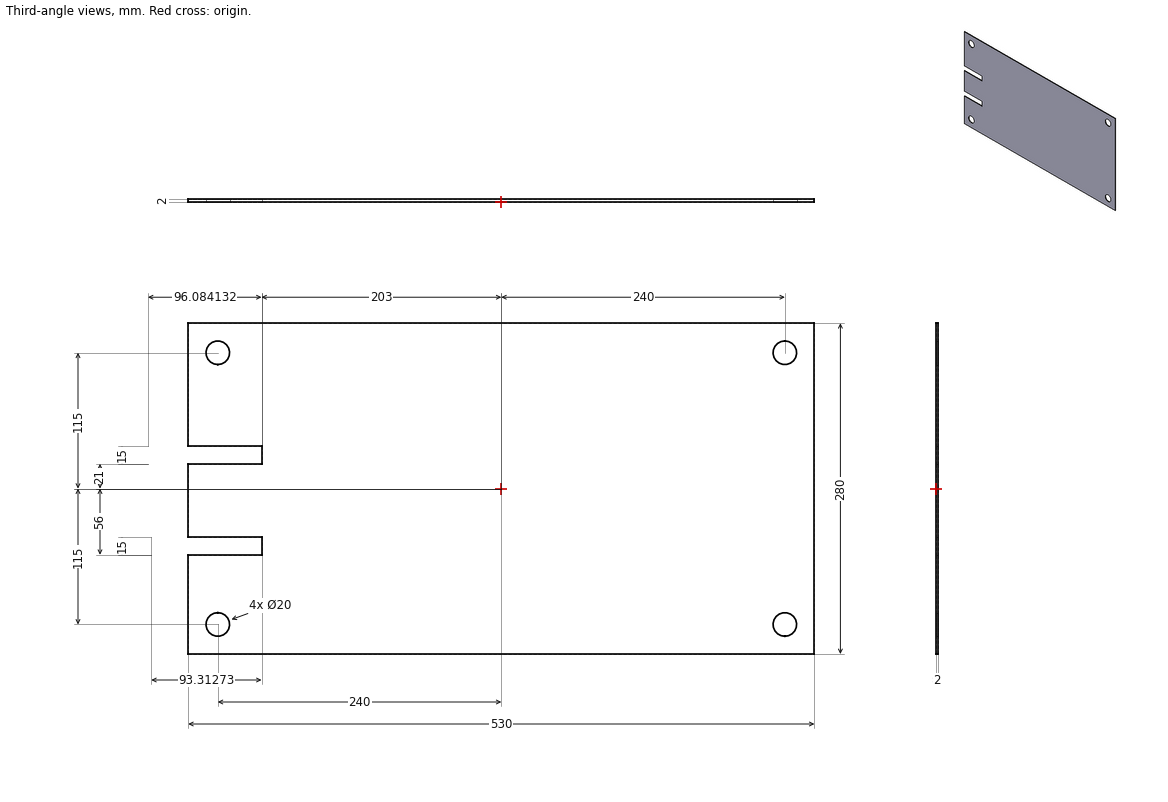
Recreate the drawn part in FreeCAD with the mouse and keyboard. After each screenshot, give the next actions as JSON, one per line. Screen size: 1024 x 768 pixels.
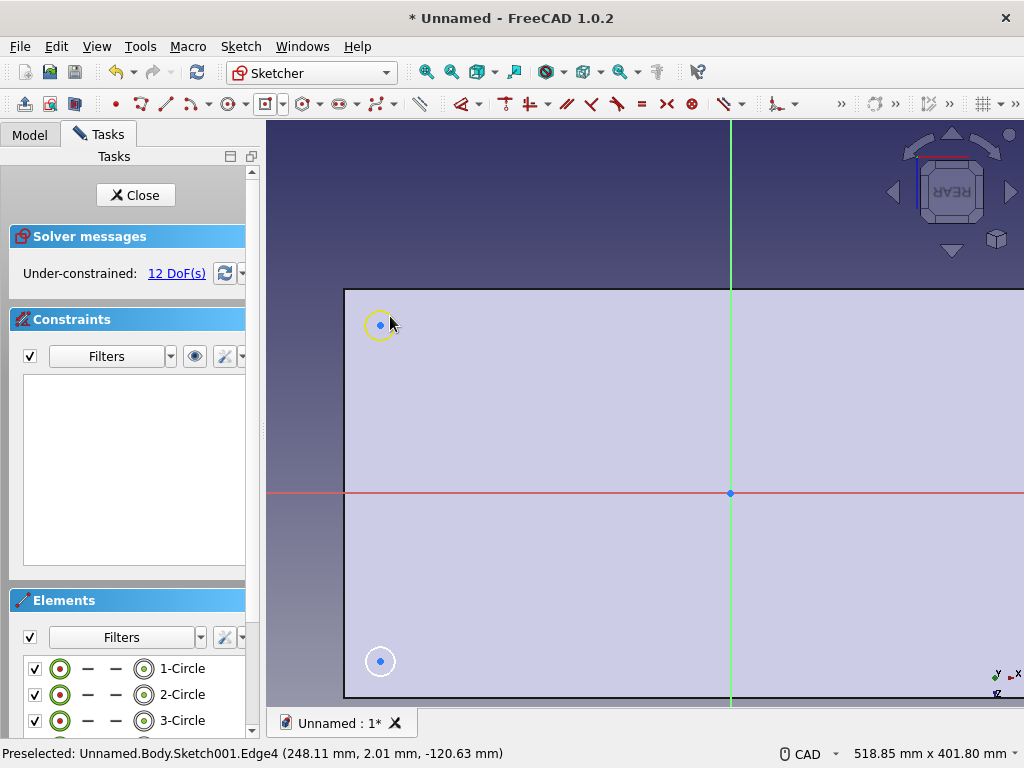
{"action": "left_click", "coordinate": [390, 315]}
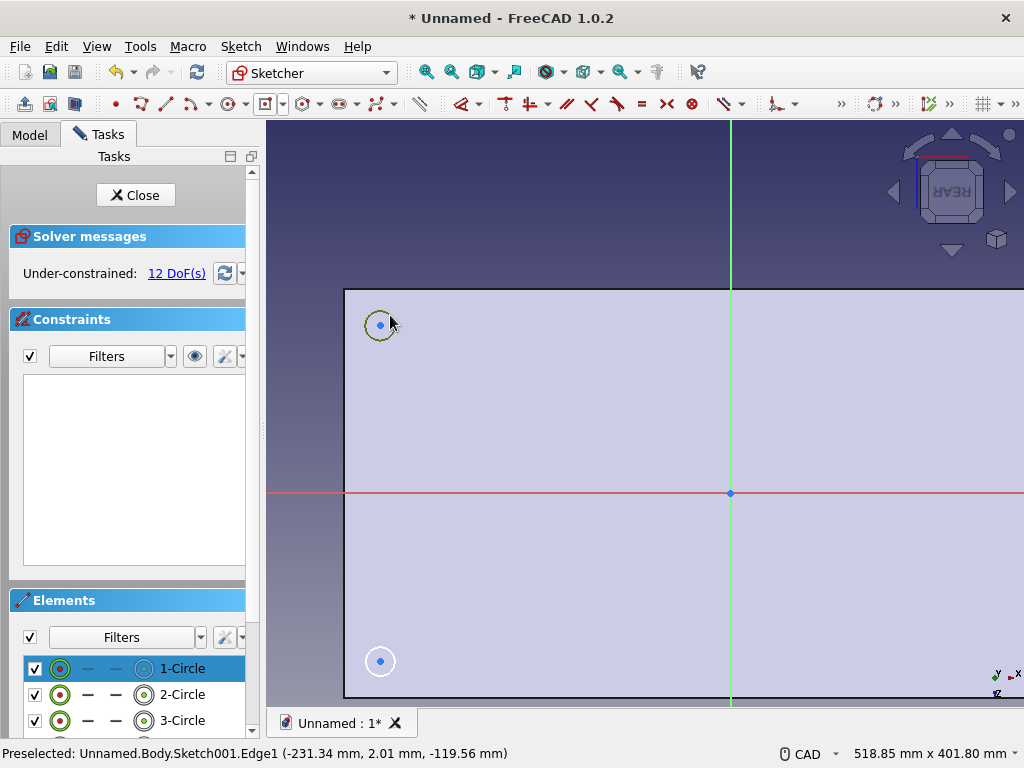
{"action": "left_click", "coordinate": [391, 651]}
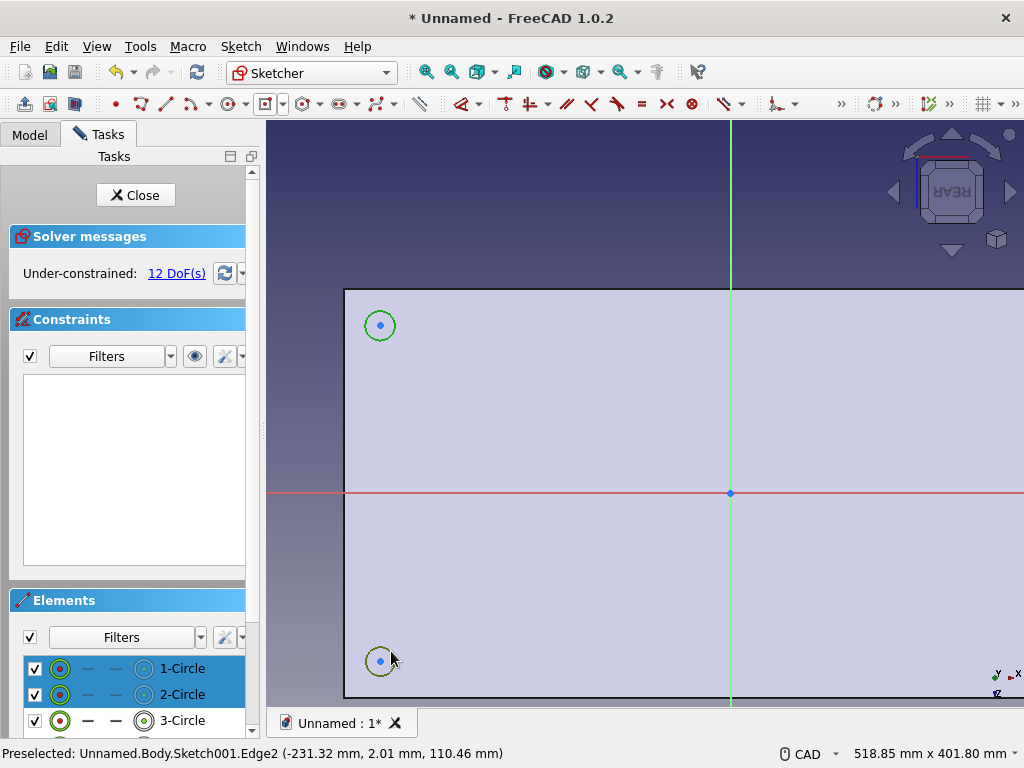
{"action": "scroll", "coordinate": [389, 316], "scroll_direction": "down", "scroll_amount": 3}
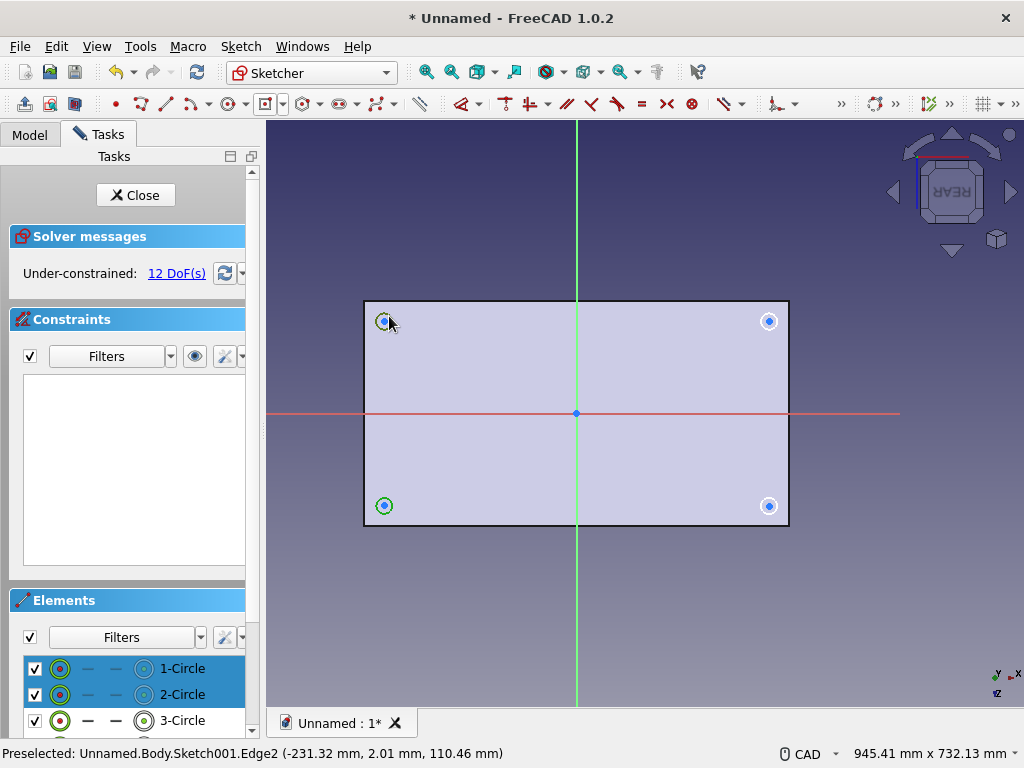
{"action": "scroll", "coordinate": [775, 500], "scroll_direction": "up", "scroll_amount": 3}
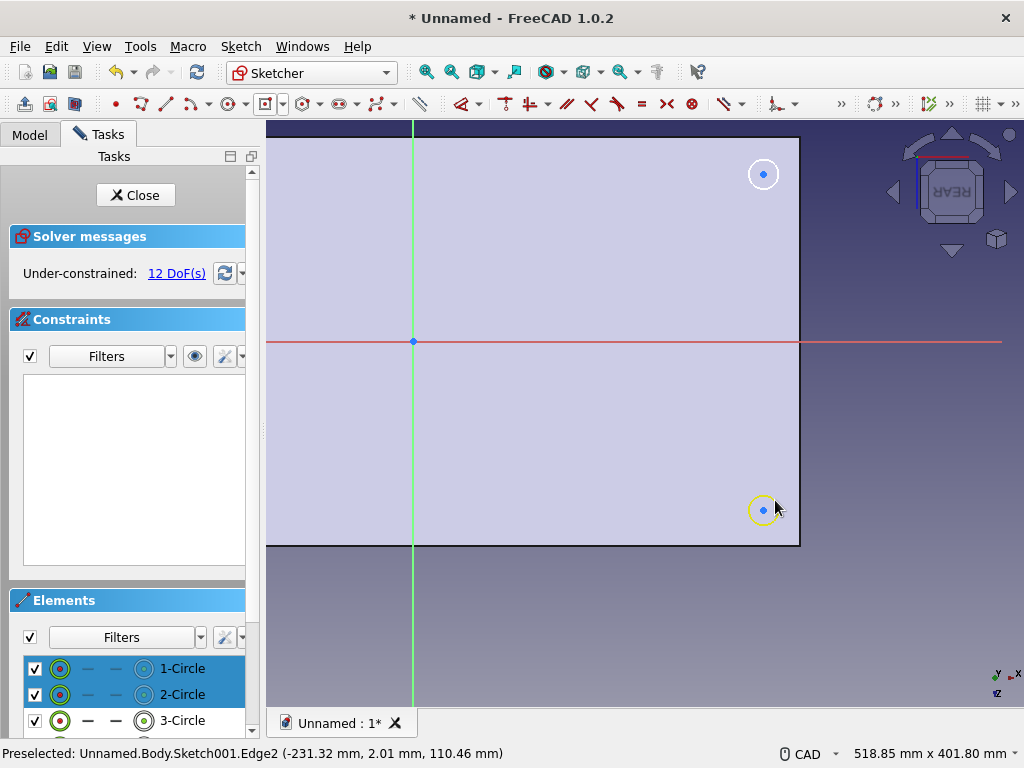
{"action": "left_click", "coordinate": [774, 500]}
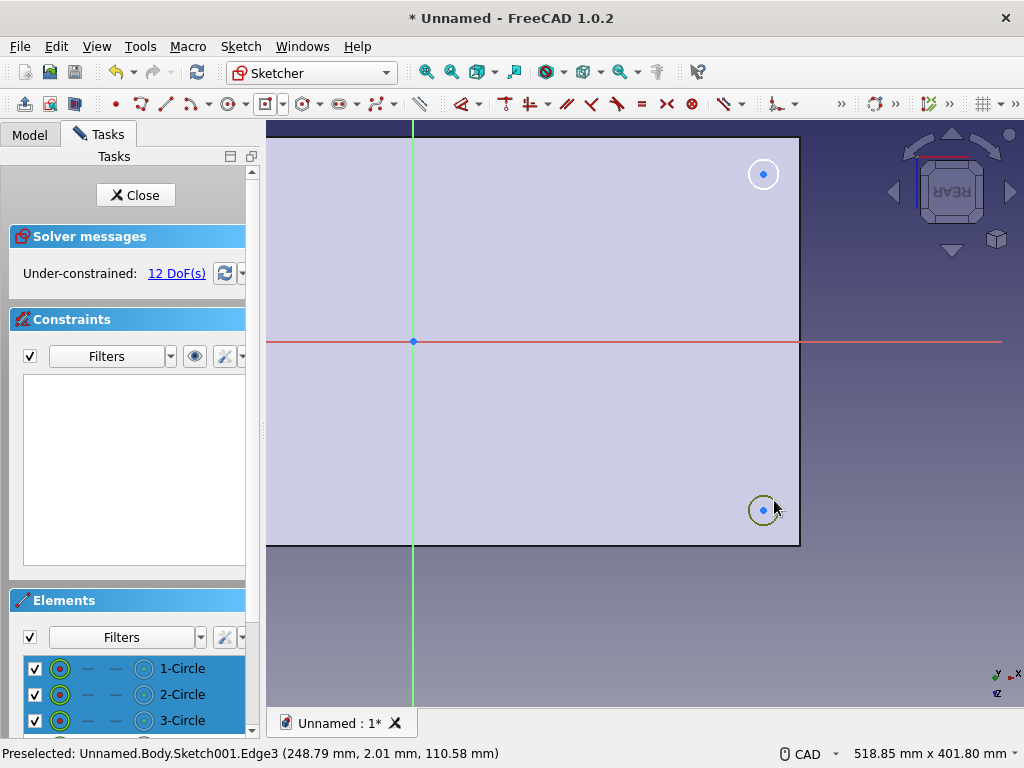
{"action": "left_click", "coordinate": [774, 164]}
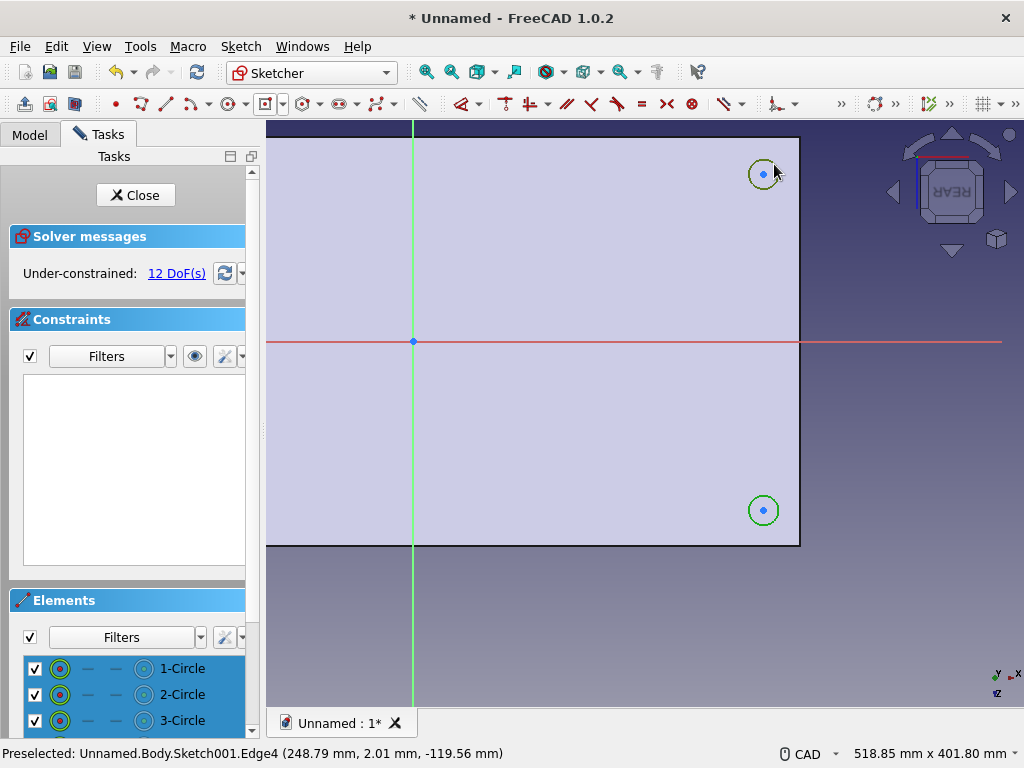
{"action": "left_click", "coordinate": [642, 104]}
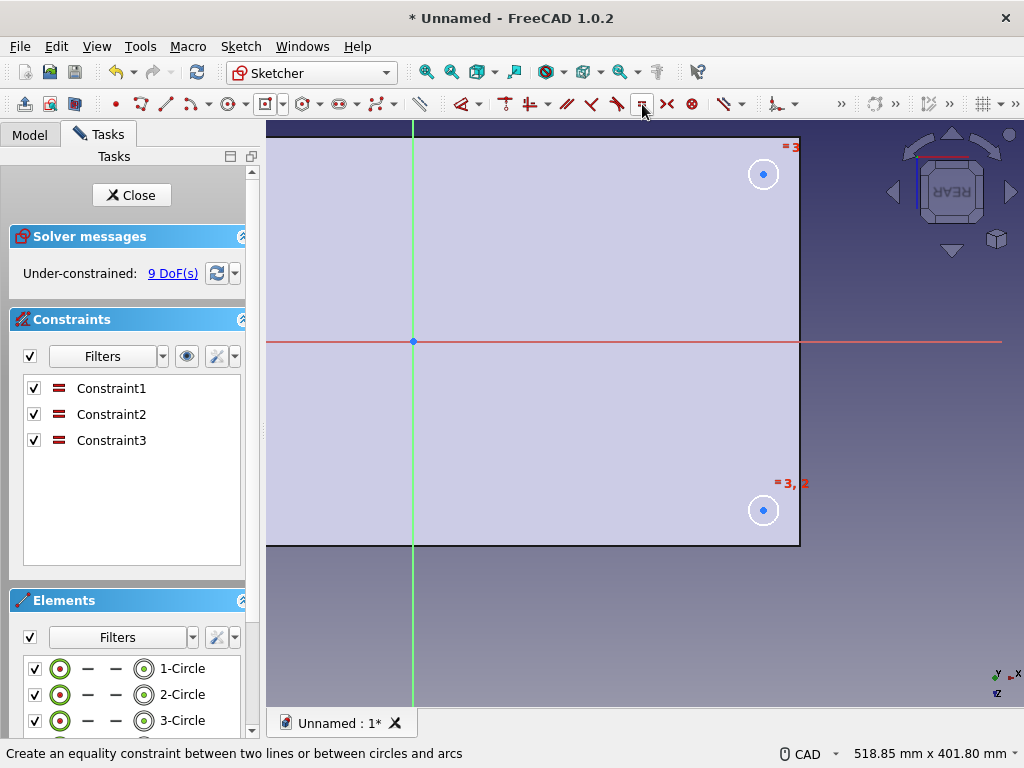
{"action": "scroll", "coordinate": [775, 501], "scroll_direction": "down", "scroll_amount": 3}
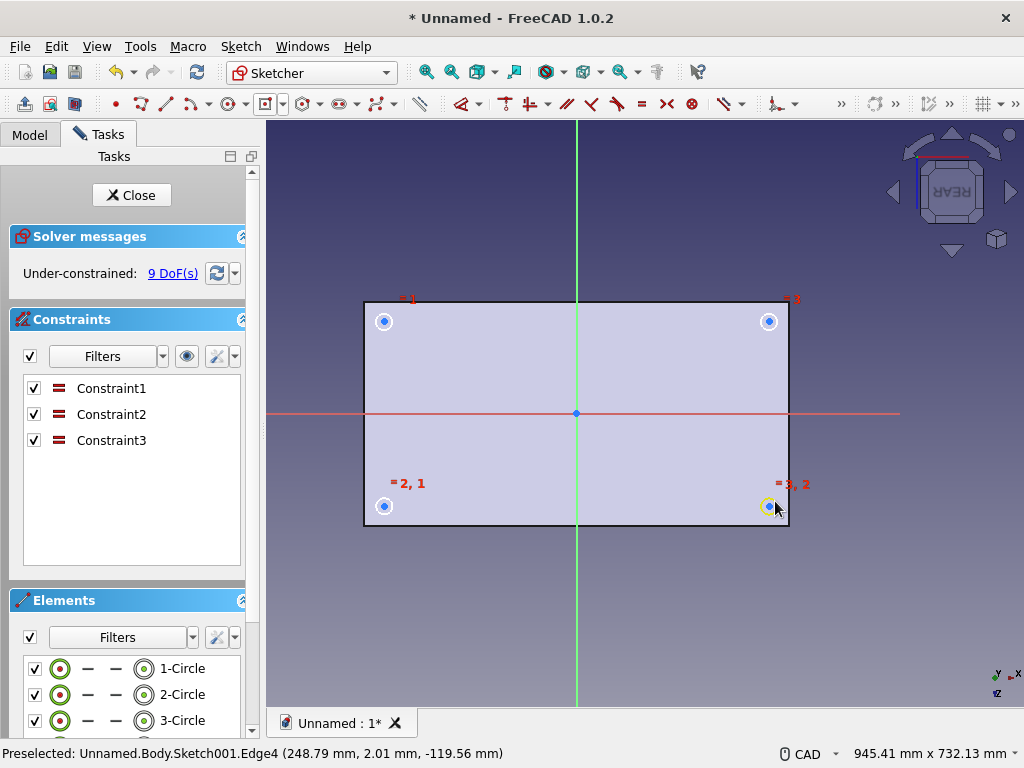
{"action": "left_click", "coordinate": [384, 322]}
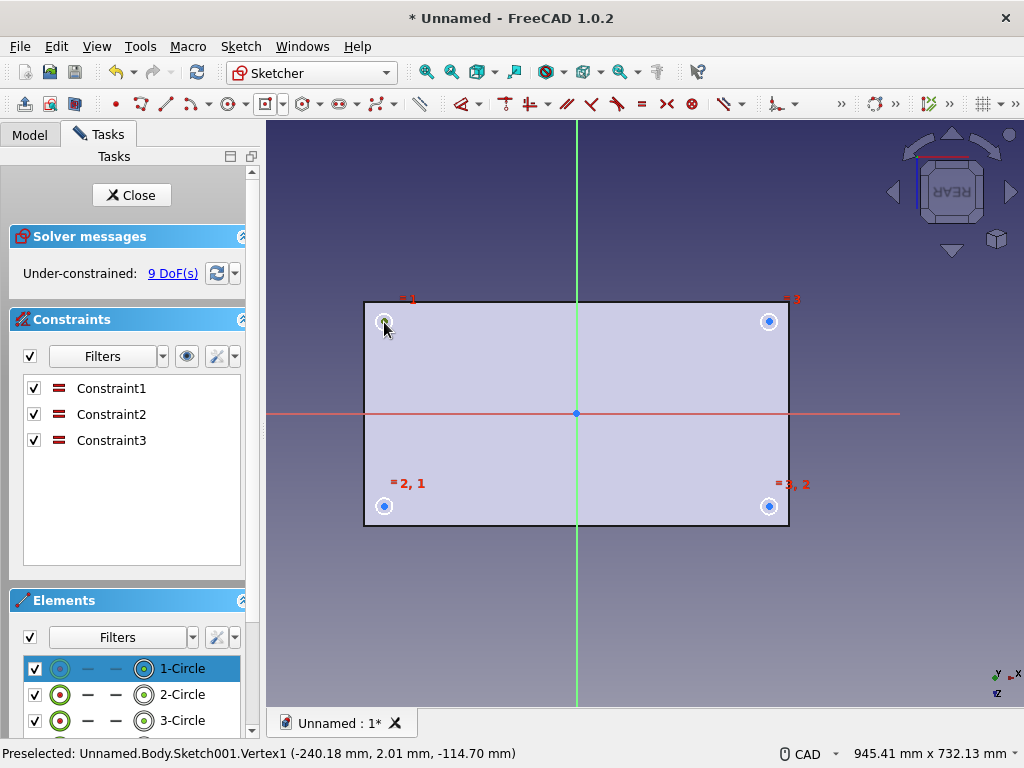
{"action": "left_click", "coordinate": [384, 506]}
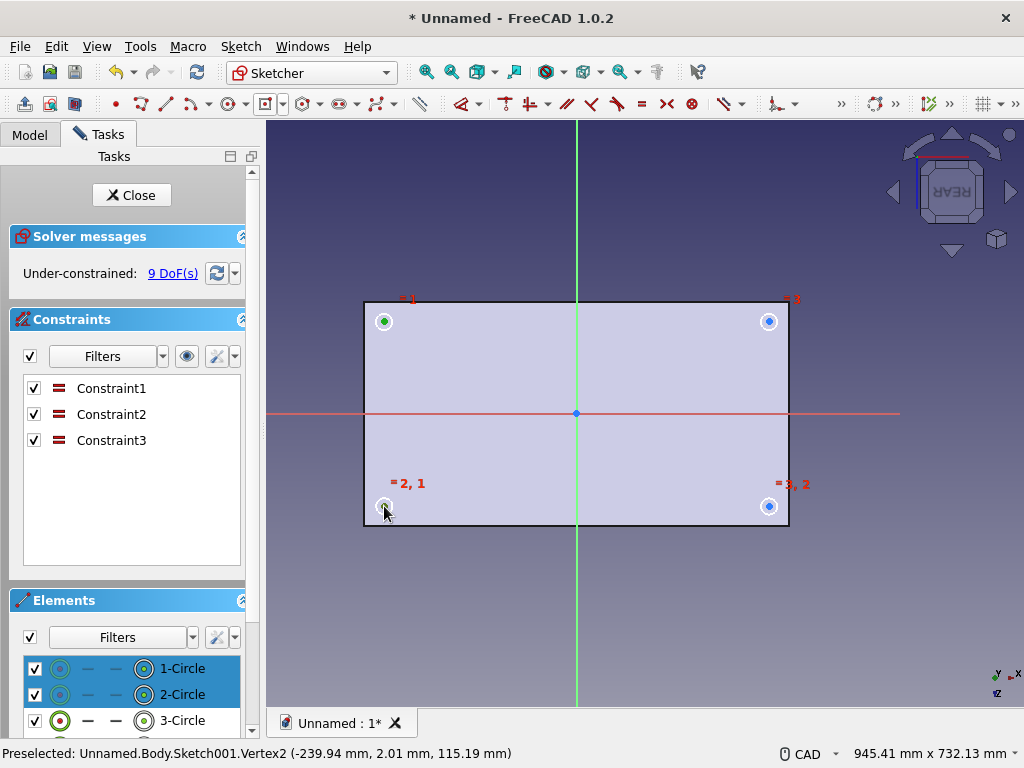
{"action": "key", "text": "v"}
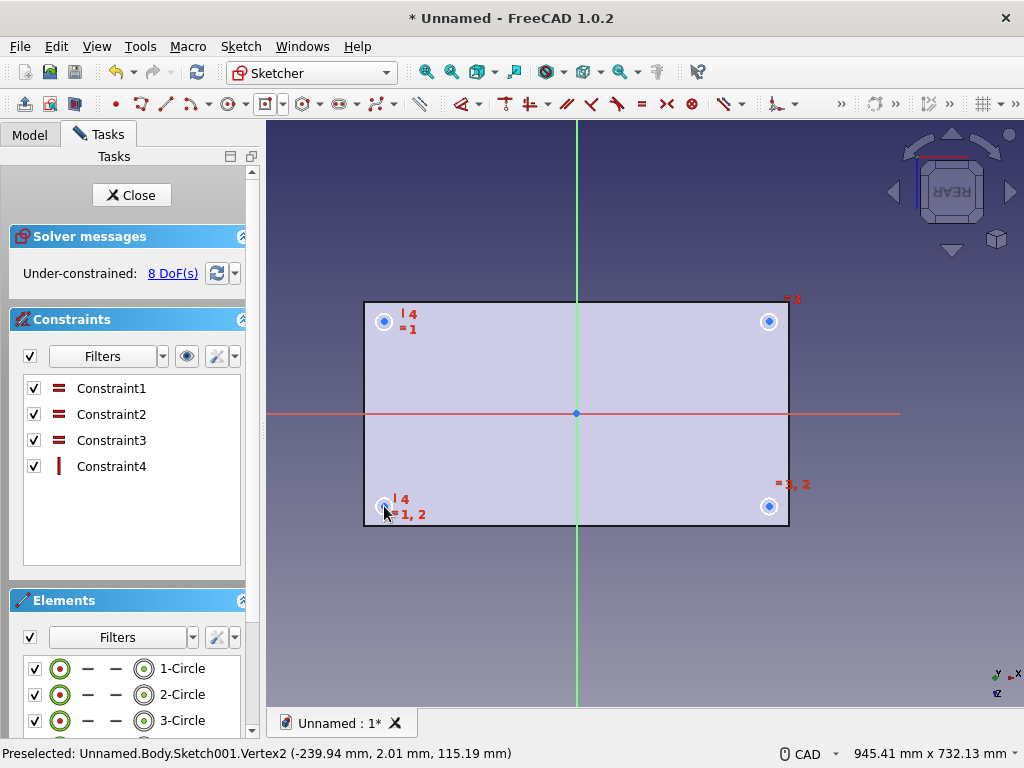
{"action": "left_click", "coordinate": [384, 506]}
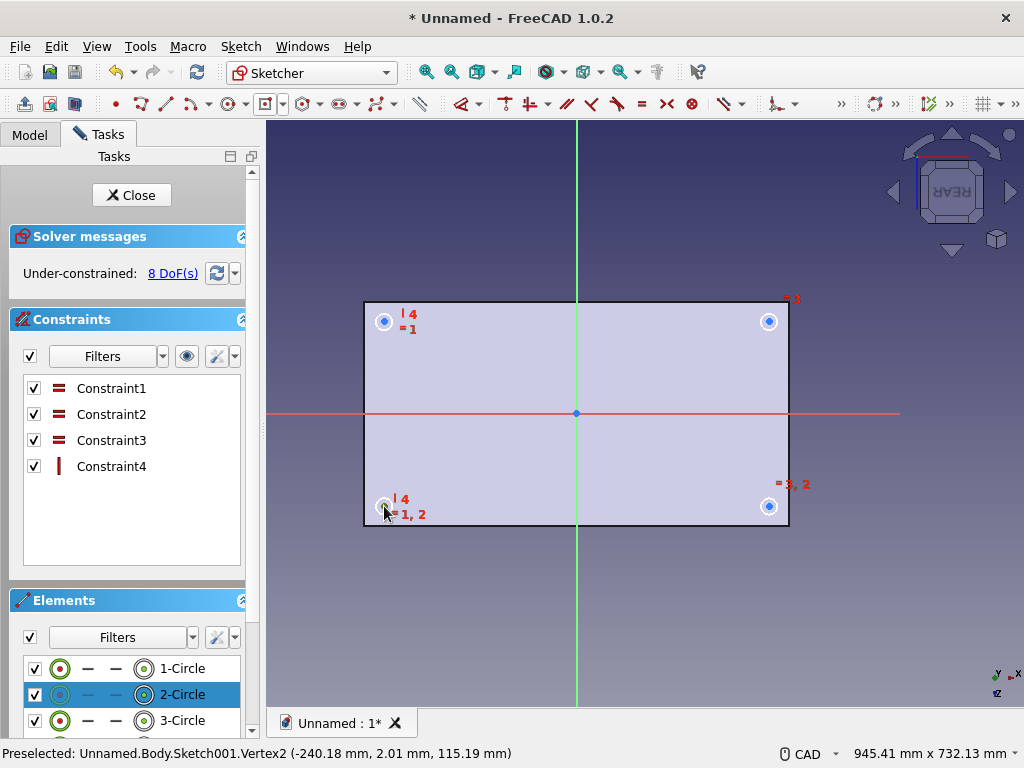
{"action": "left_click", "coordinate": [769, 507]}